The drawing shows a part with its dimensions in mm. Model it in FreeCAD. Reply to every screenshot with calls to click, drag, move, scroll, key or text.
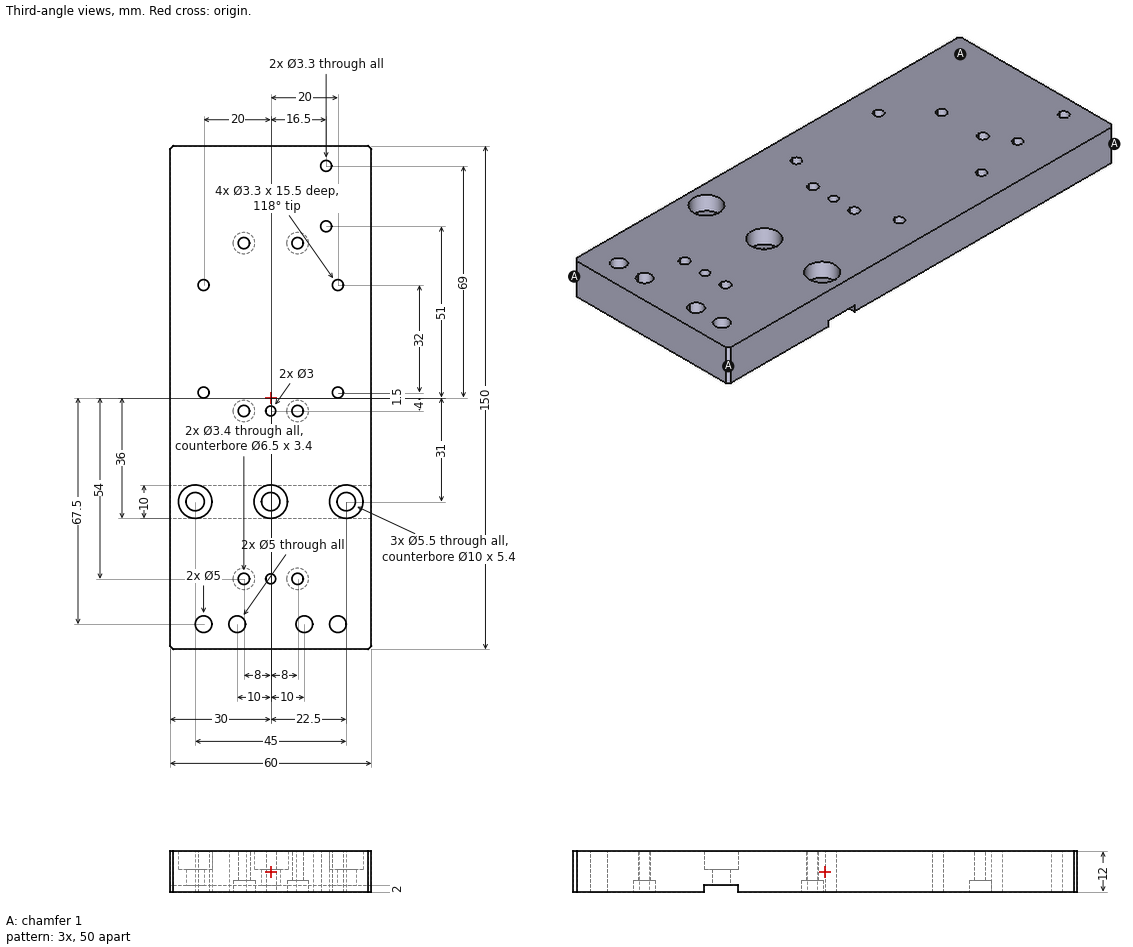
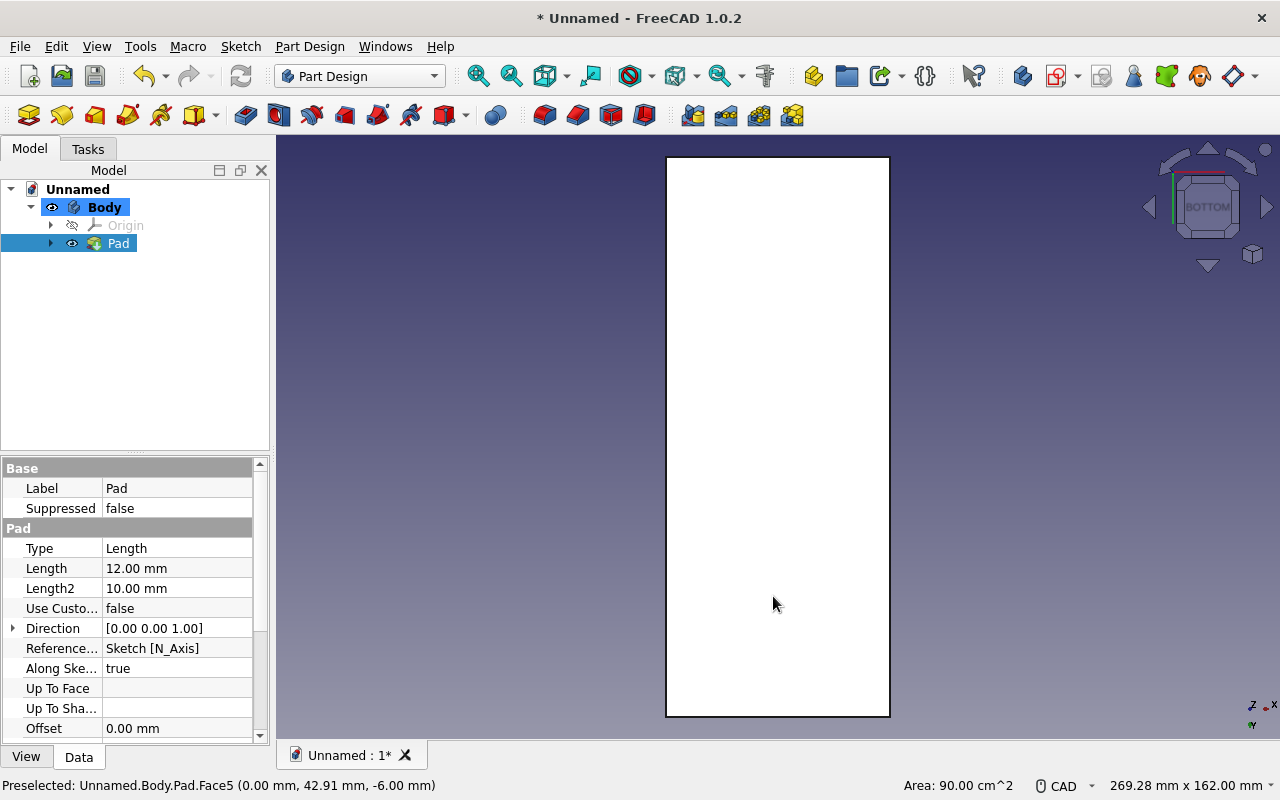
click(1056, 76)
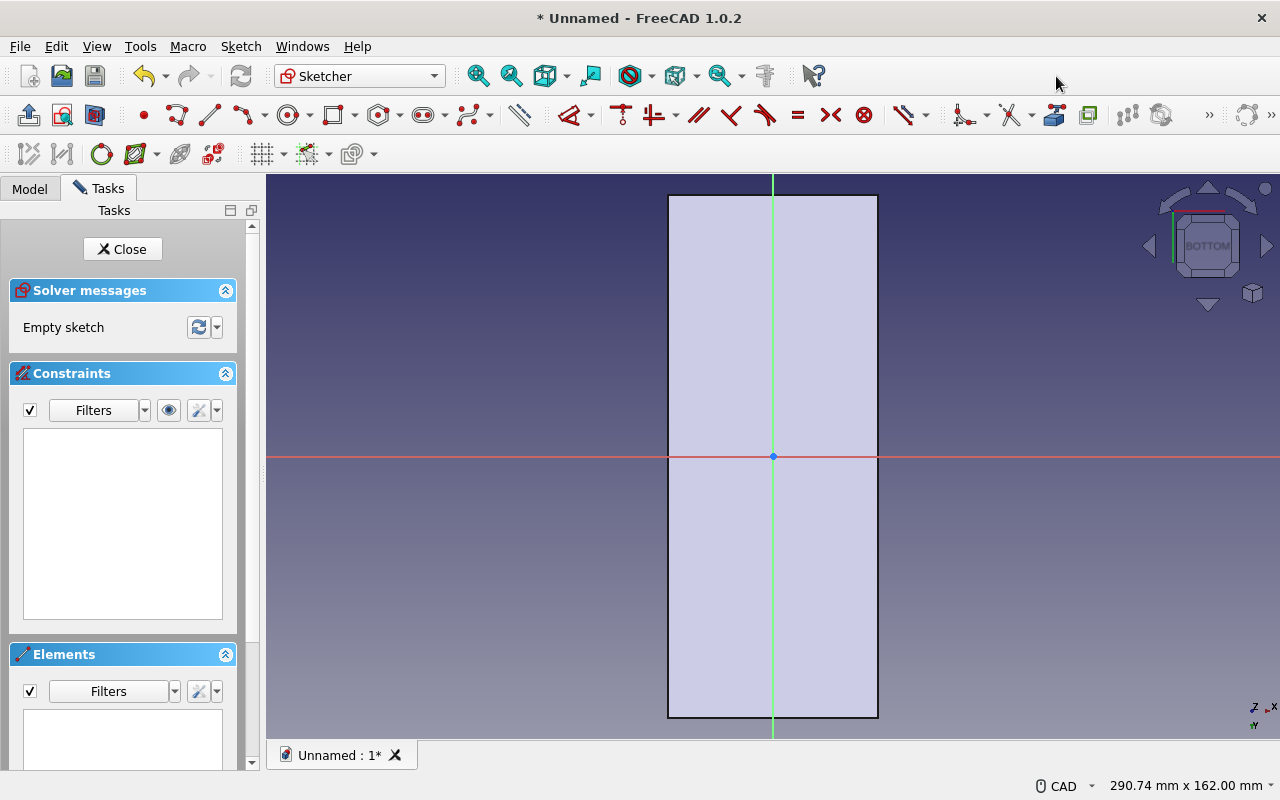
scroll(862, 711, up, 8)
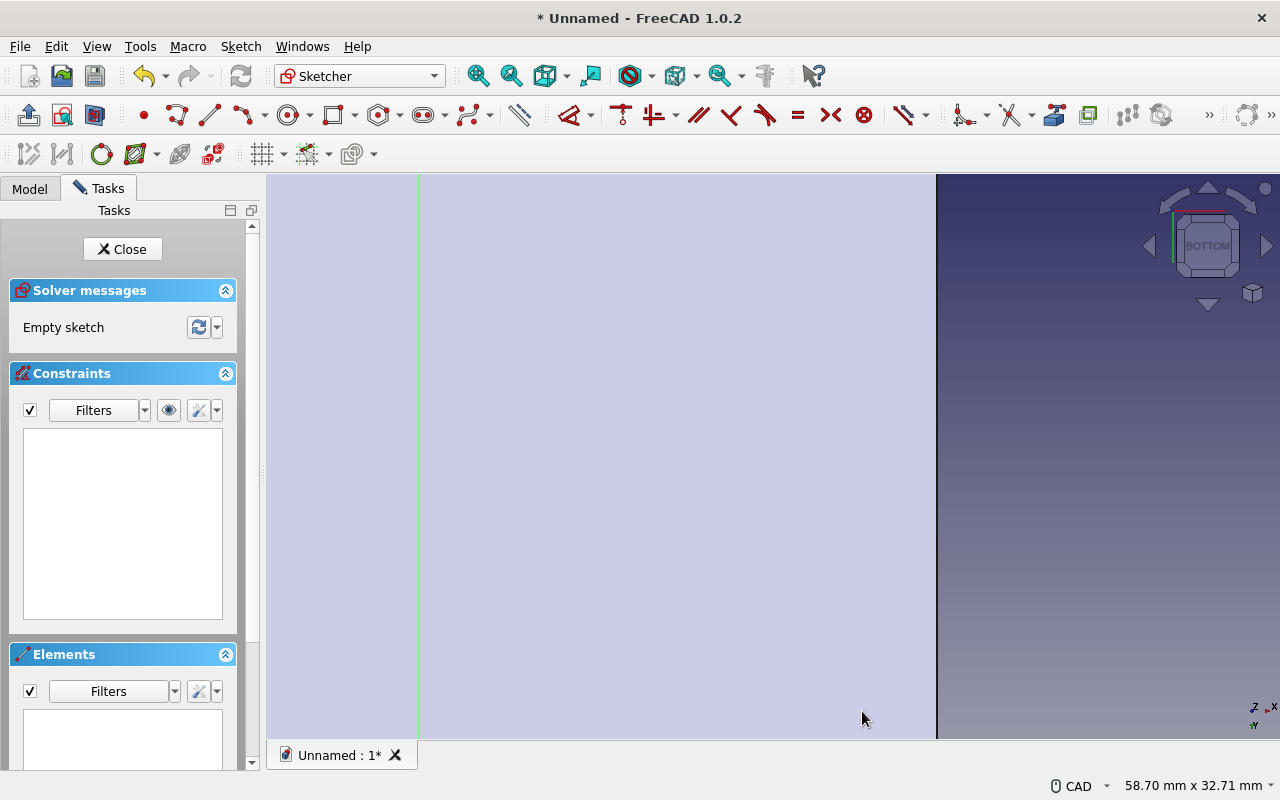
click(288, 116)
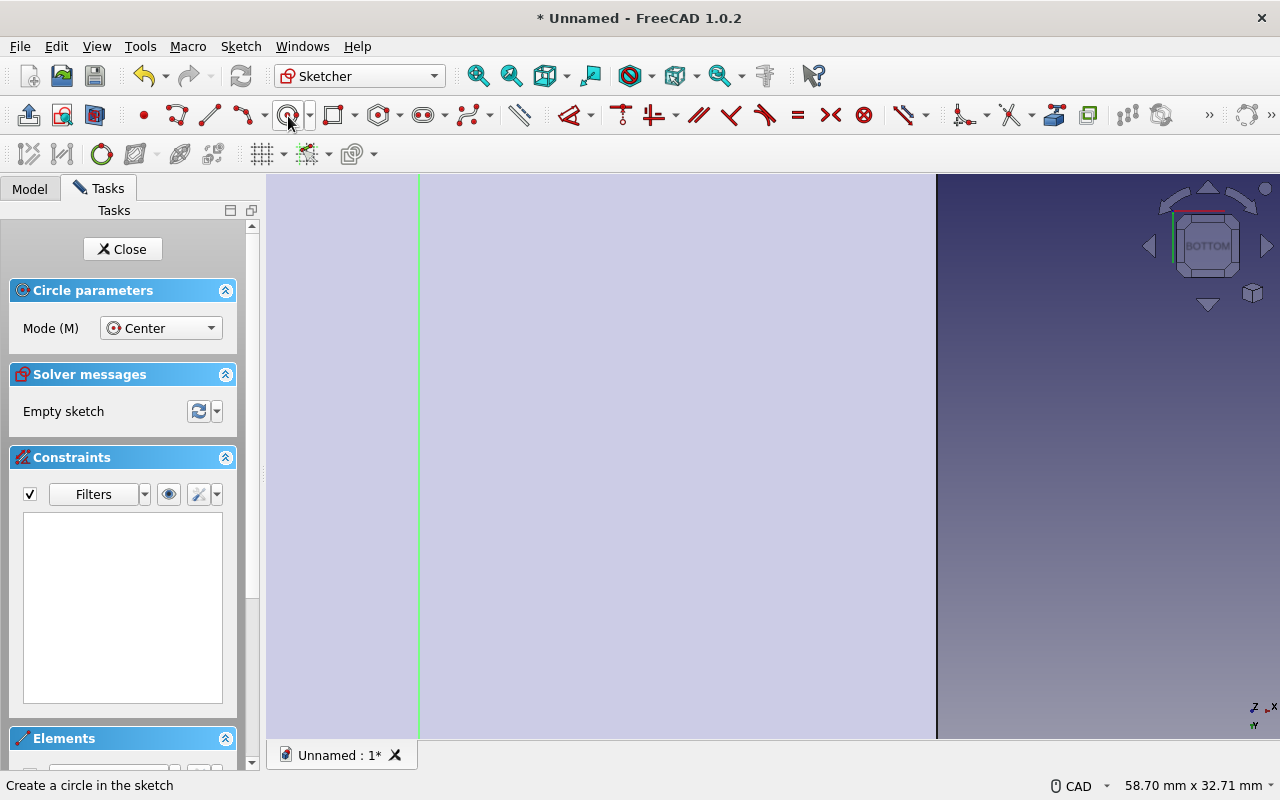
click(704, 639)
click(724, 618)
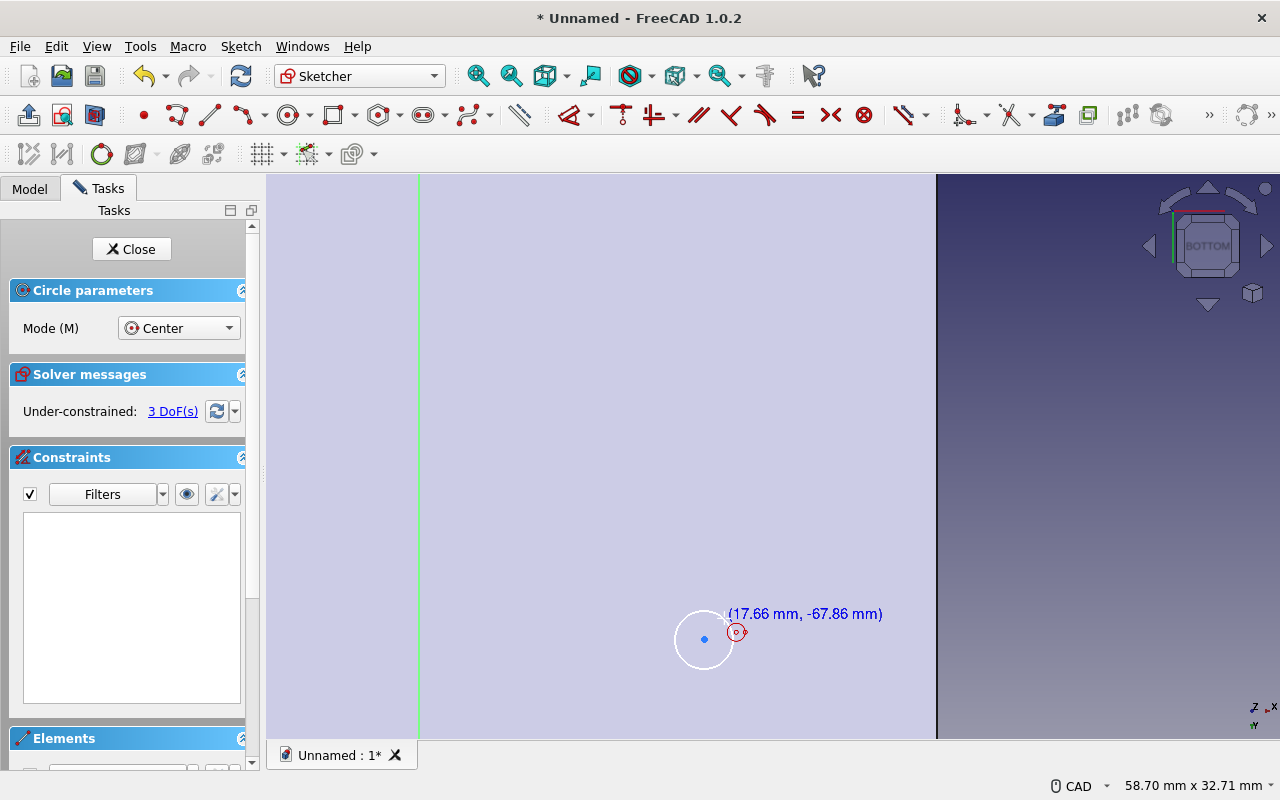
click(704, 328)
click(724, 308)
key(Escape)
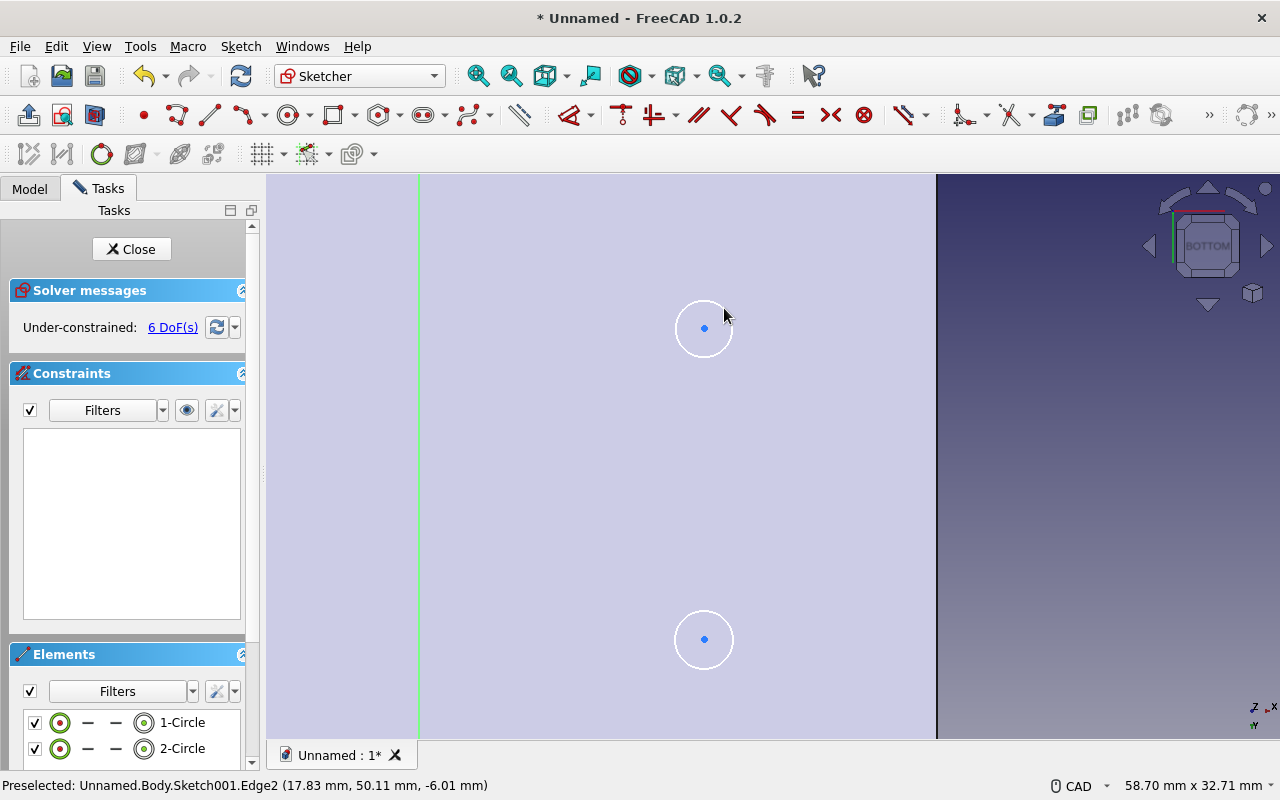
click(724, 619)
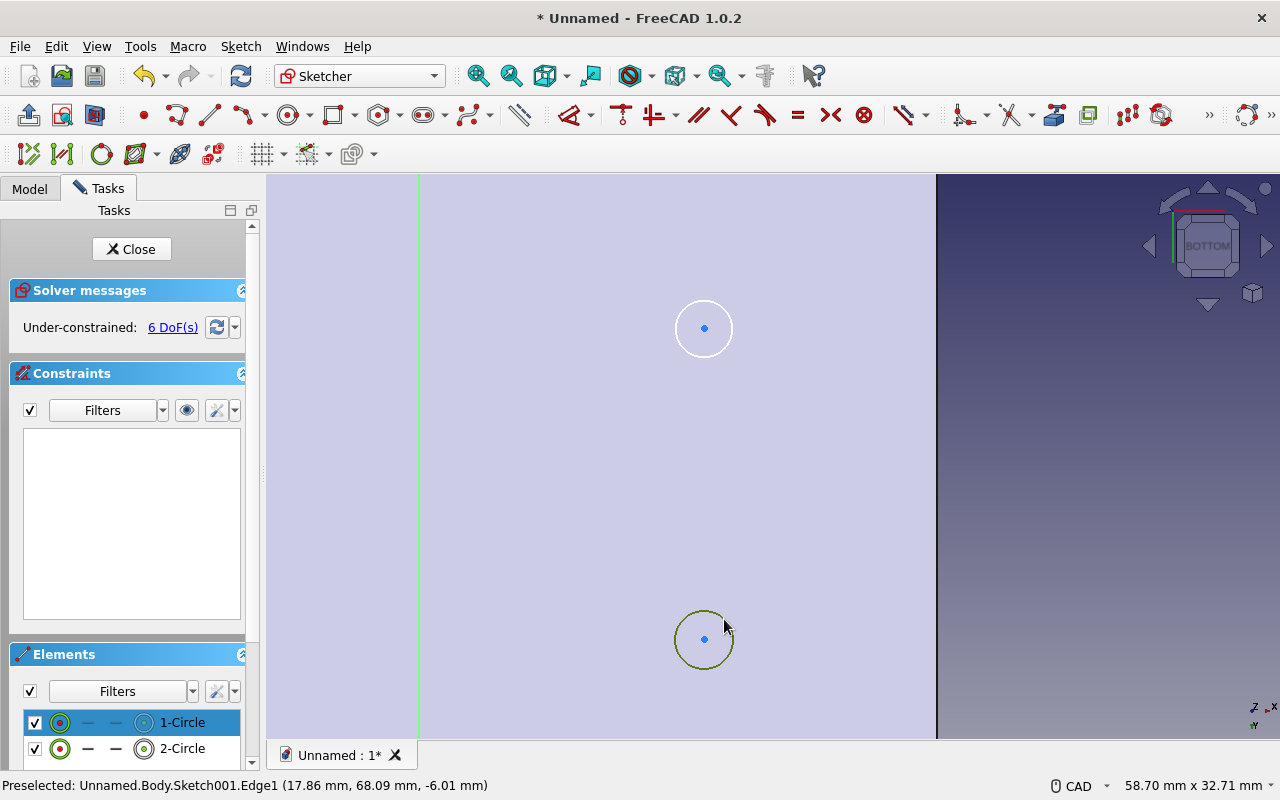
click(724, 309)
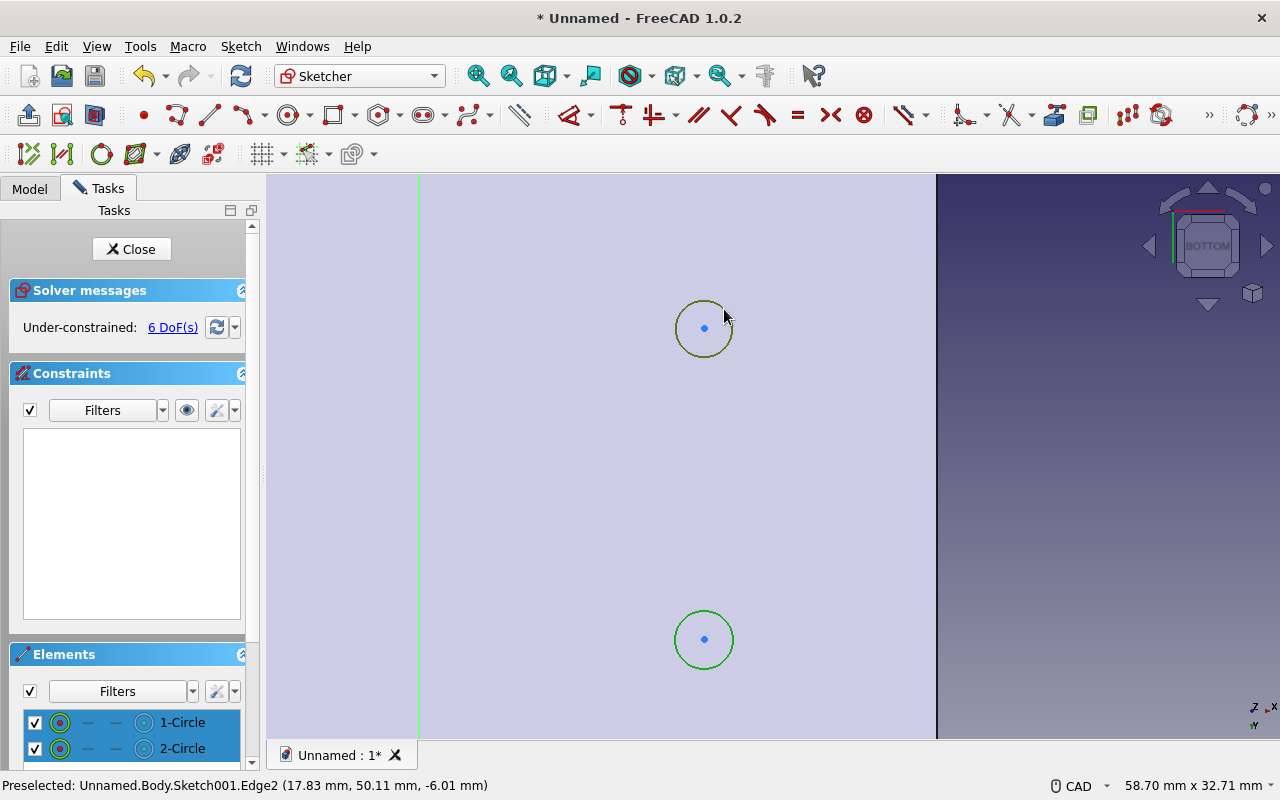
click(798, 116)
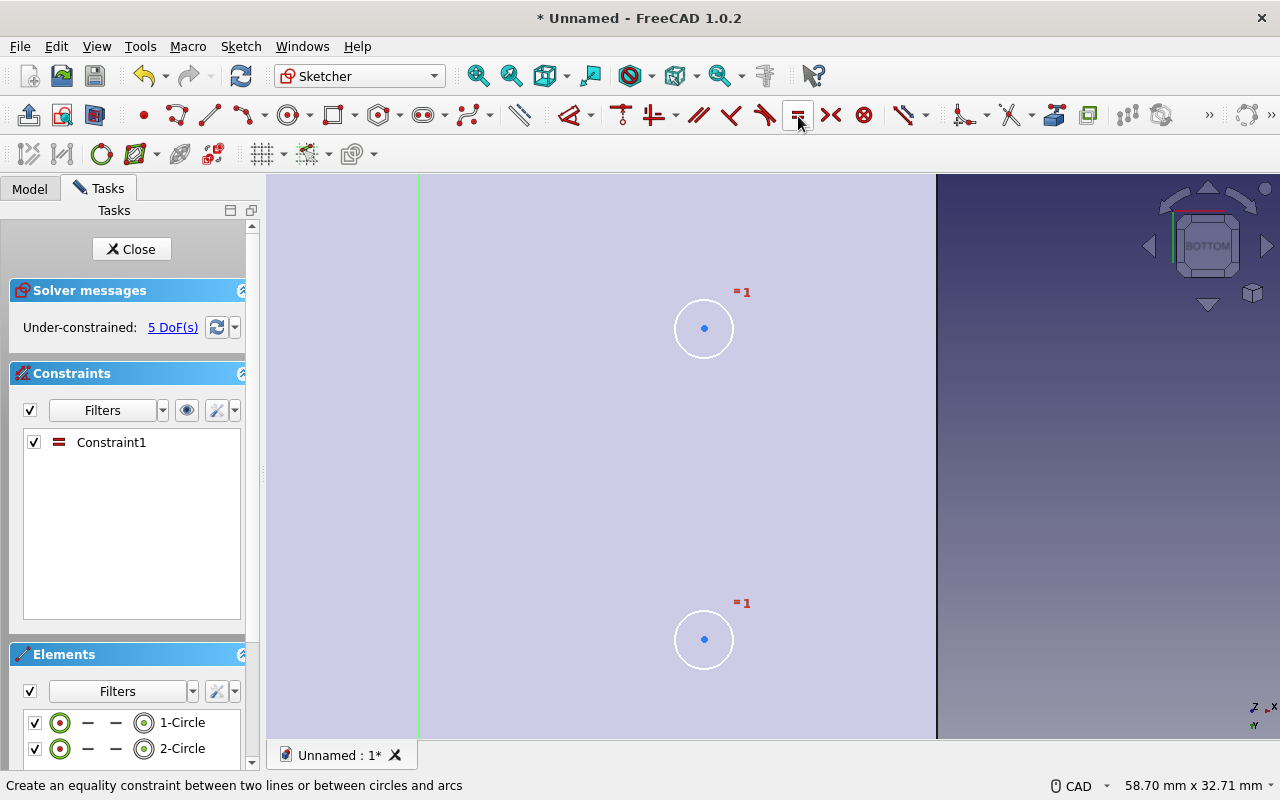
click(704, 640)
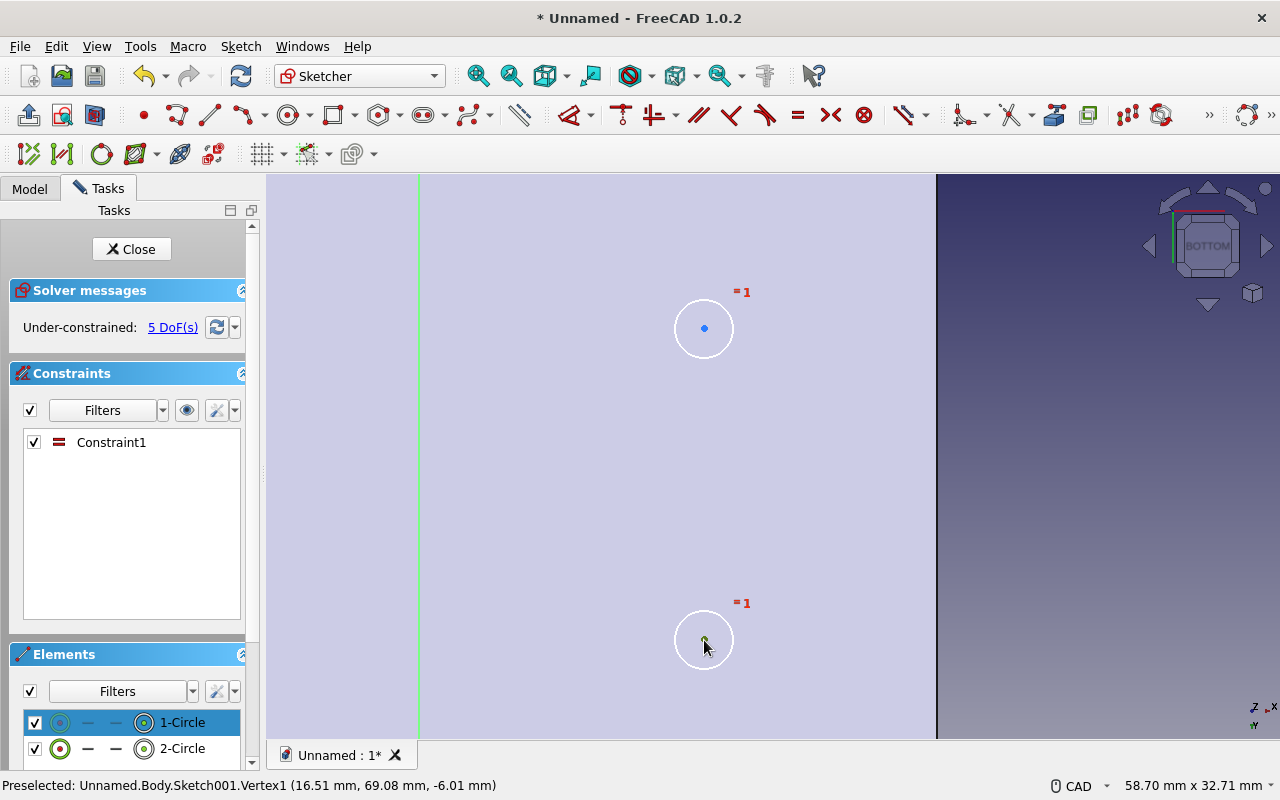
click(704, 329)